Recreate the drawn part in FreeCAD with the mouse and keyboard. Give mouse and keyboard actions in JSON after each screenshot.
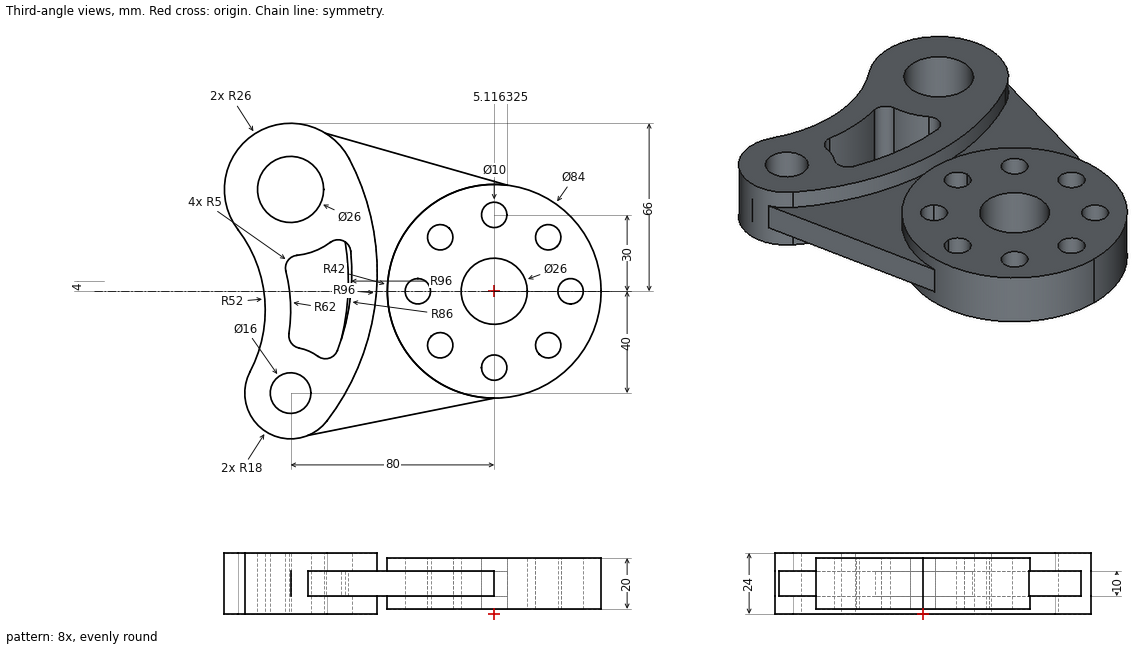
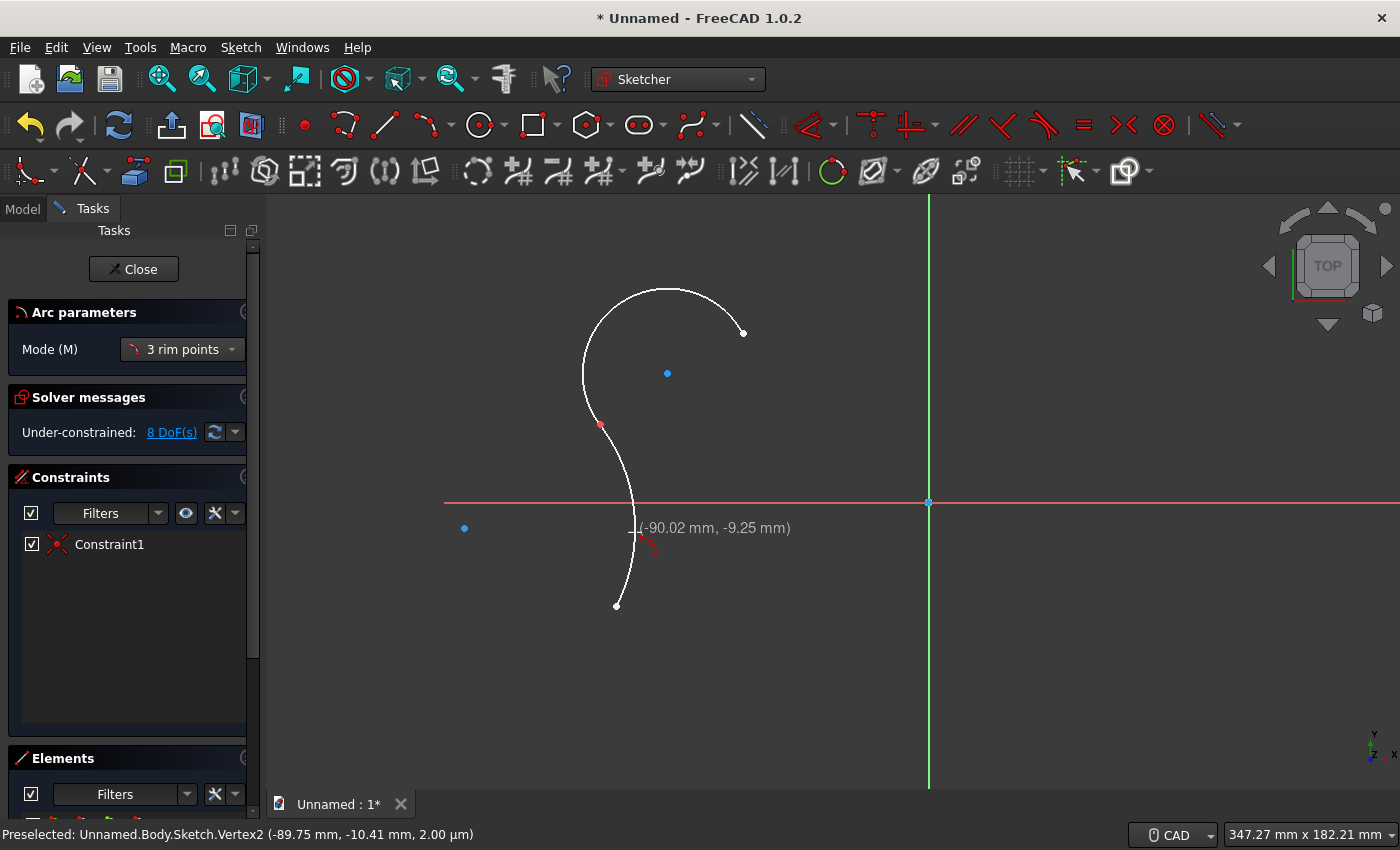
{"action": "left_click", "coordinate": [616, 607]}
{"action": "left_click", "coordinate": [714, 669]}
{"action": "left_click", "coordinate": [636, 683]}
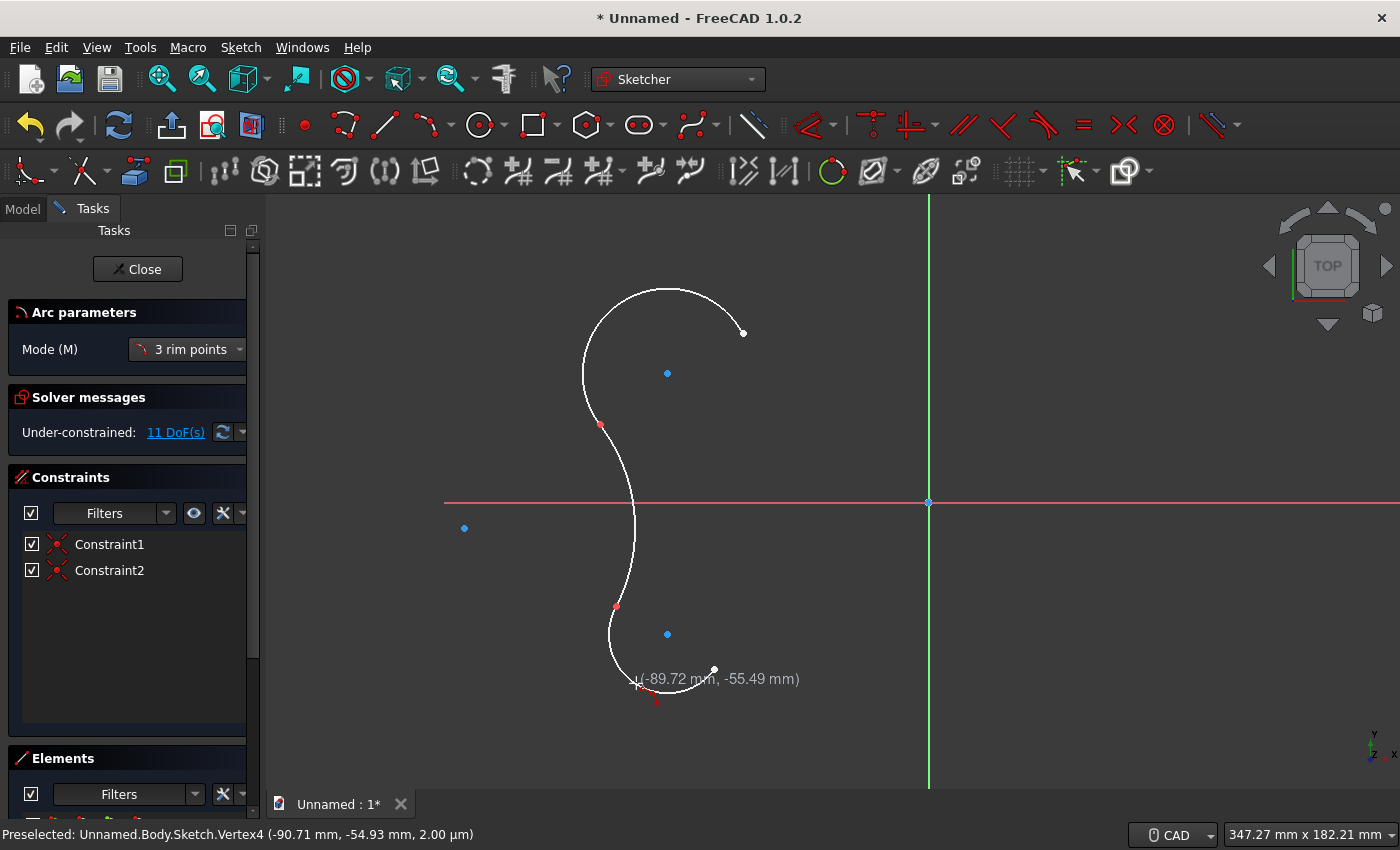
{"action": "left_click", "coordinate": [714, 670]}
{"action": "left_click", "coordinate": [743, 334]}
{"action": "left_click", "coordinate": [773, 540]}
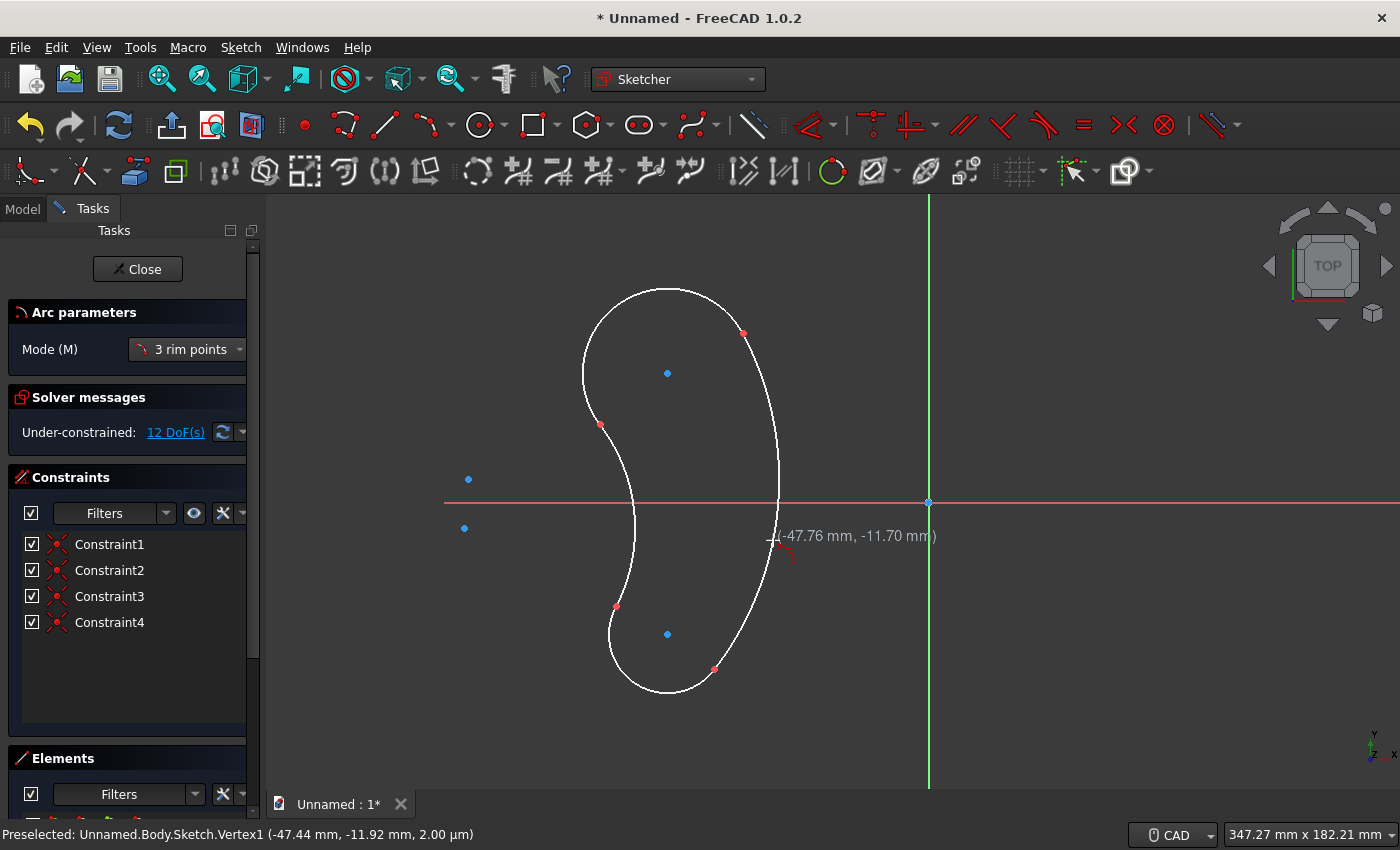
{"action": "left_click", "coordinate": [745, 451]}
{"action": "left_click", "coordinate": [728, 579]}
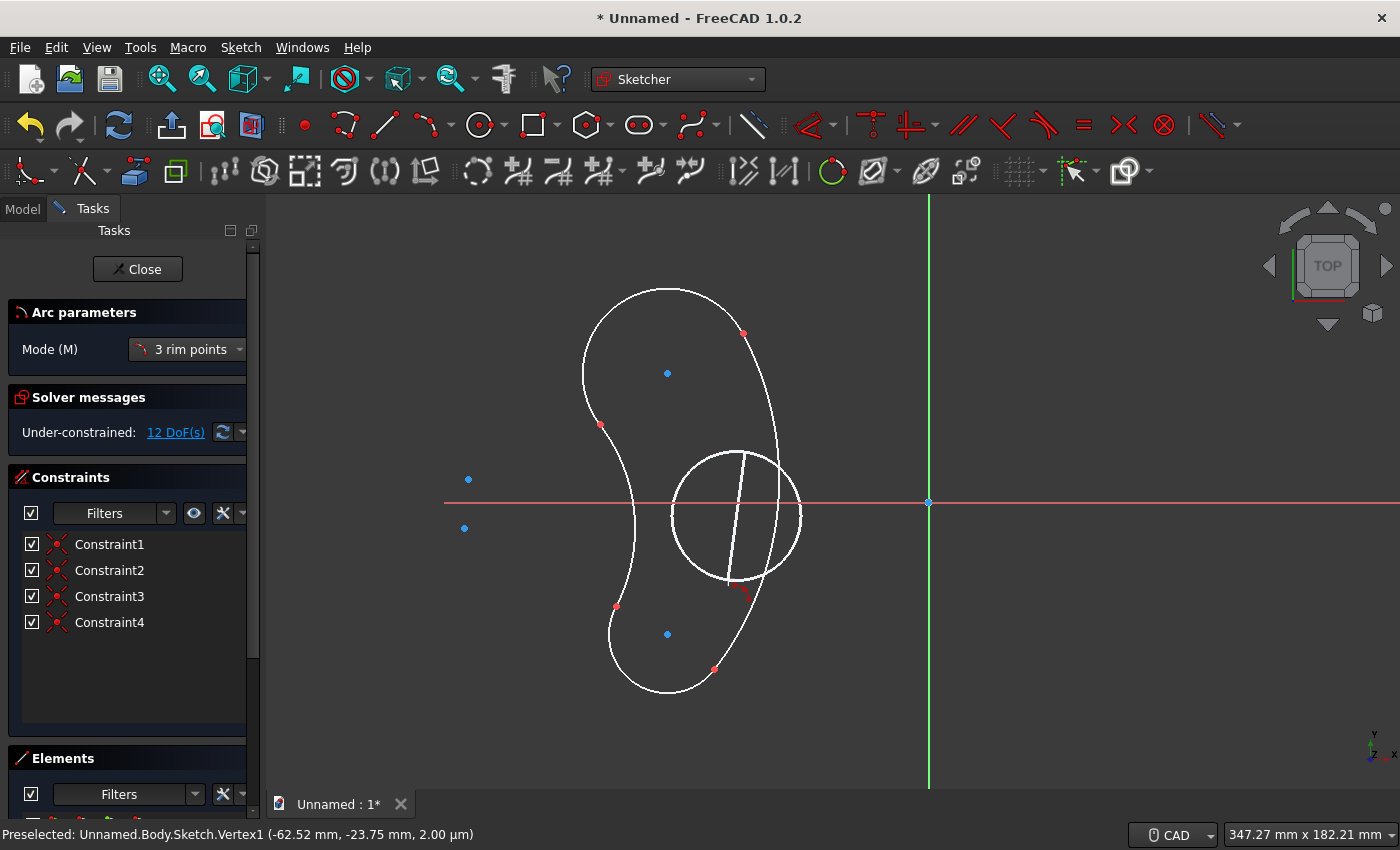
{"action": "scroll", "coordinate": [744, 516], "scroll_direction": "up", "scroll_amount": 4}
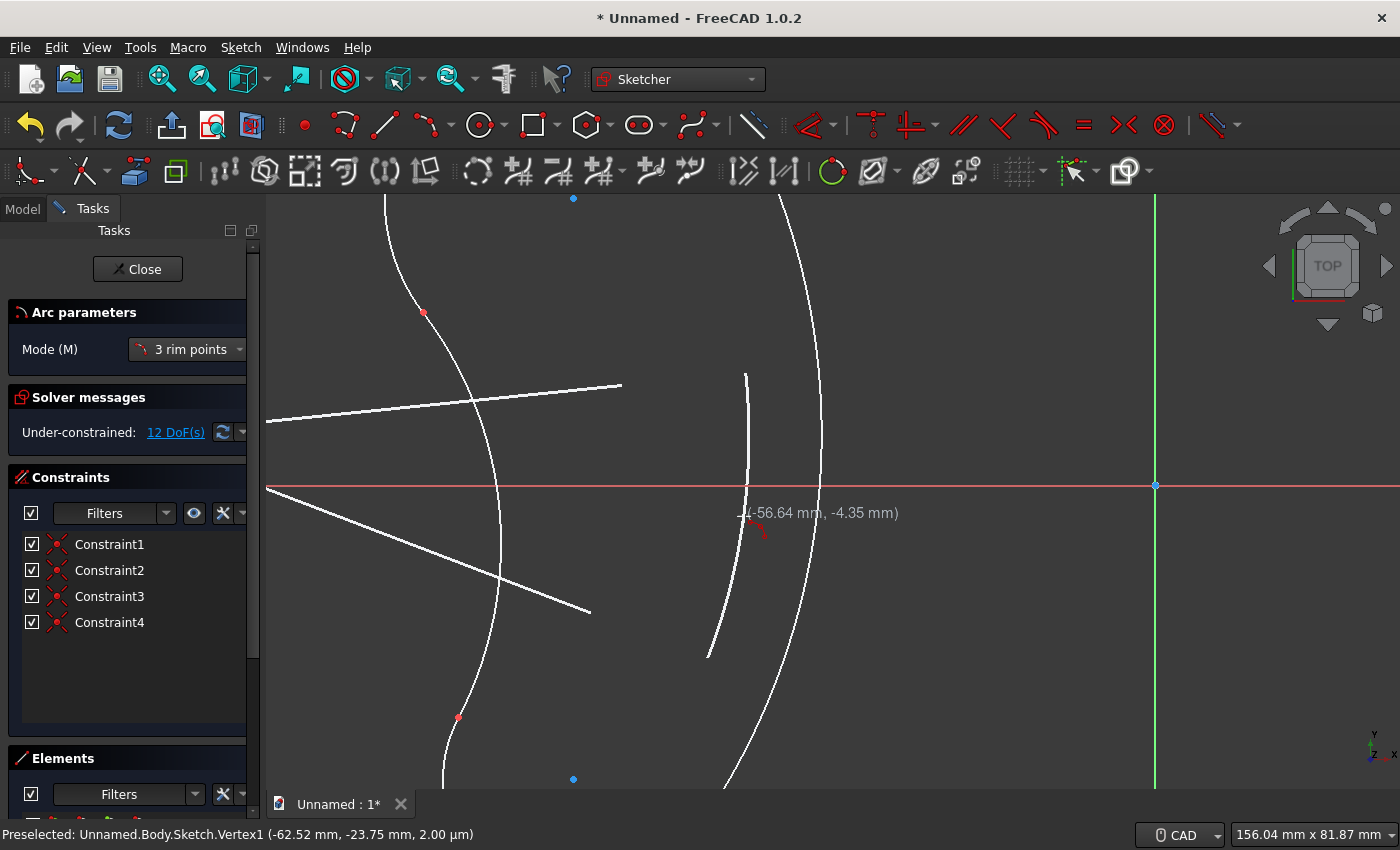
{"action": "left_click", "coordinate": [743, 516]}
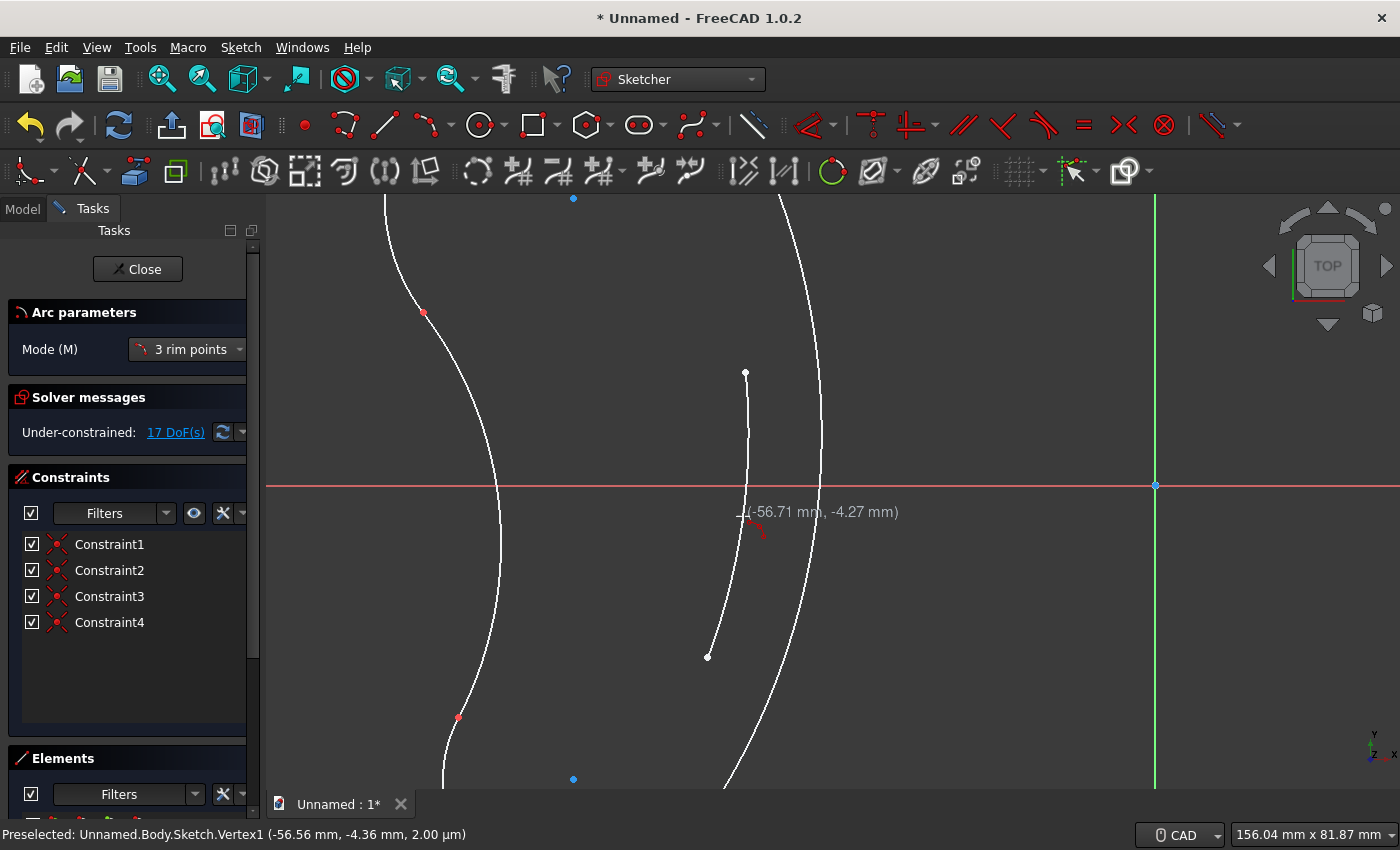
{"action": "left_click", "coordinate": [708, 658]}
{"action": "left_click", "coordinate": [652, 672]}
{"action": "left_click", "coordinate": [684, 677]}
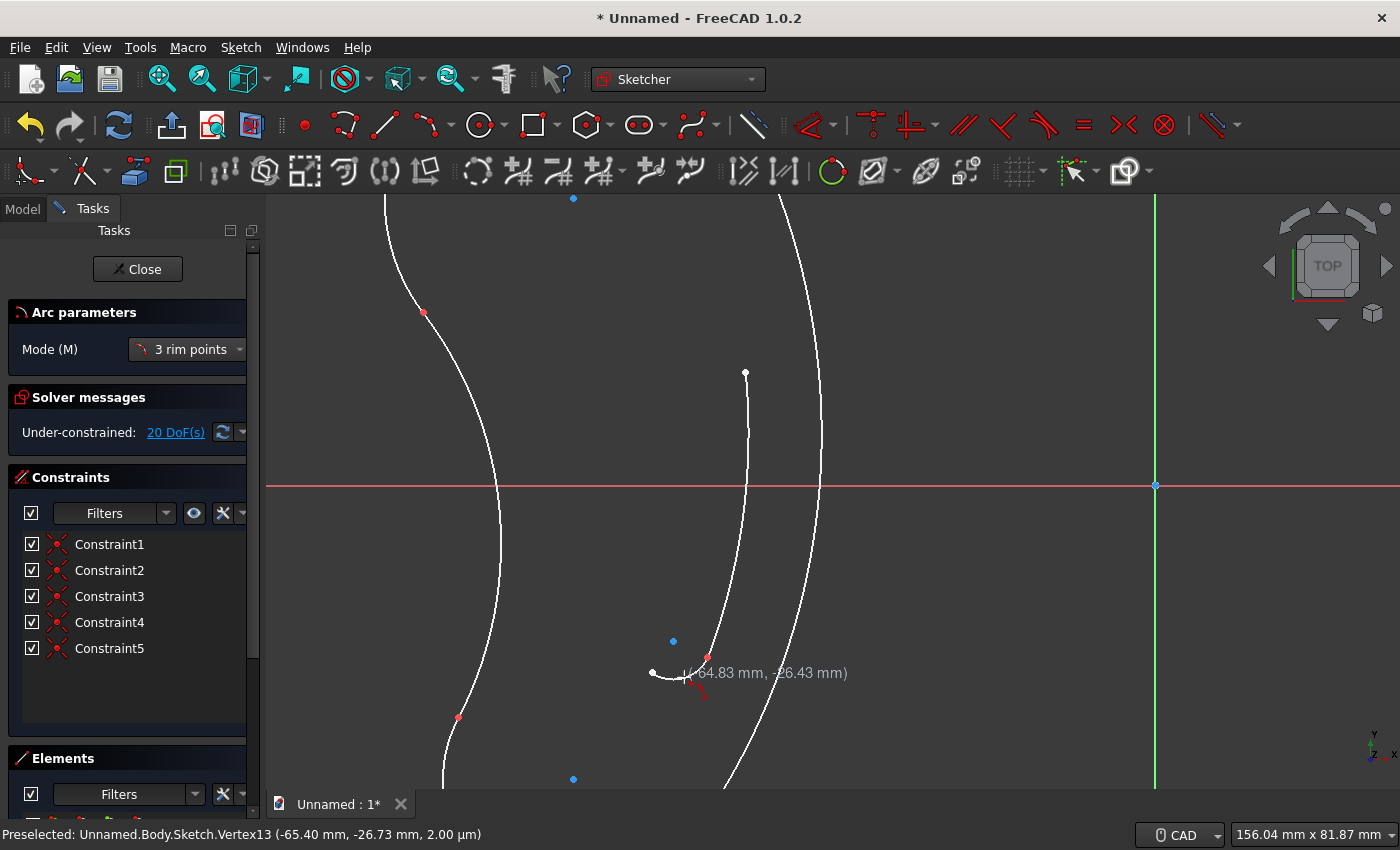
{"action": "left_click", "coordinate": [652, 673]}
{"action": "left_click", "coordinate": [598, 648]}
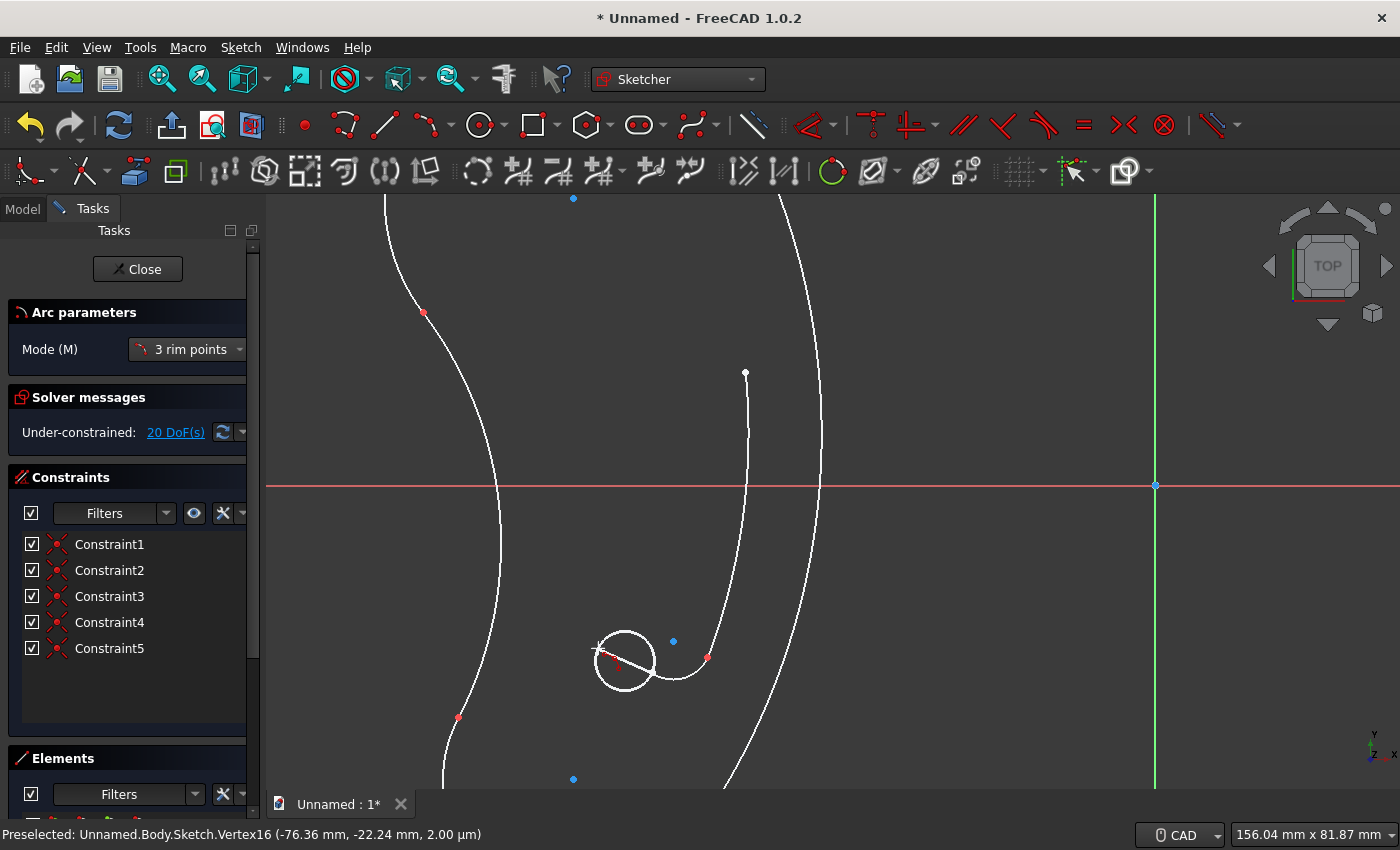
{"action": "scroll", "coordinate": [626, 657], "scroll_direction": "up", "scroll_amount": 8}